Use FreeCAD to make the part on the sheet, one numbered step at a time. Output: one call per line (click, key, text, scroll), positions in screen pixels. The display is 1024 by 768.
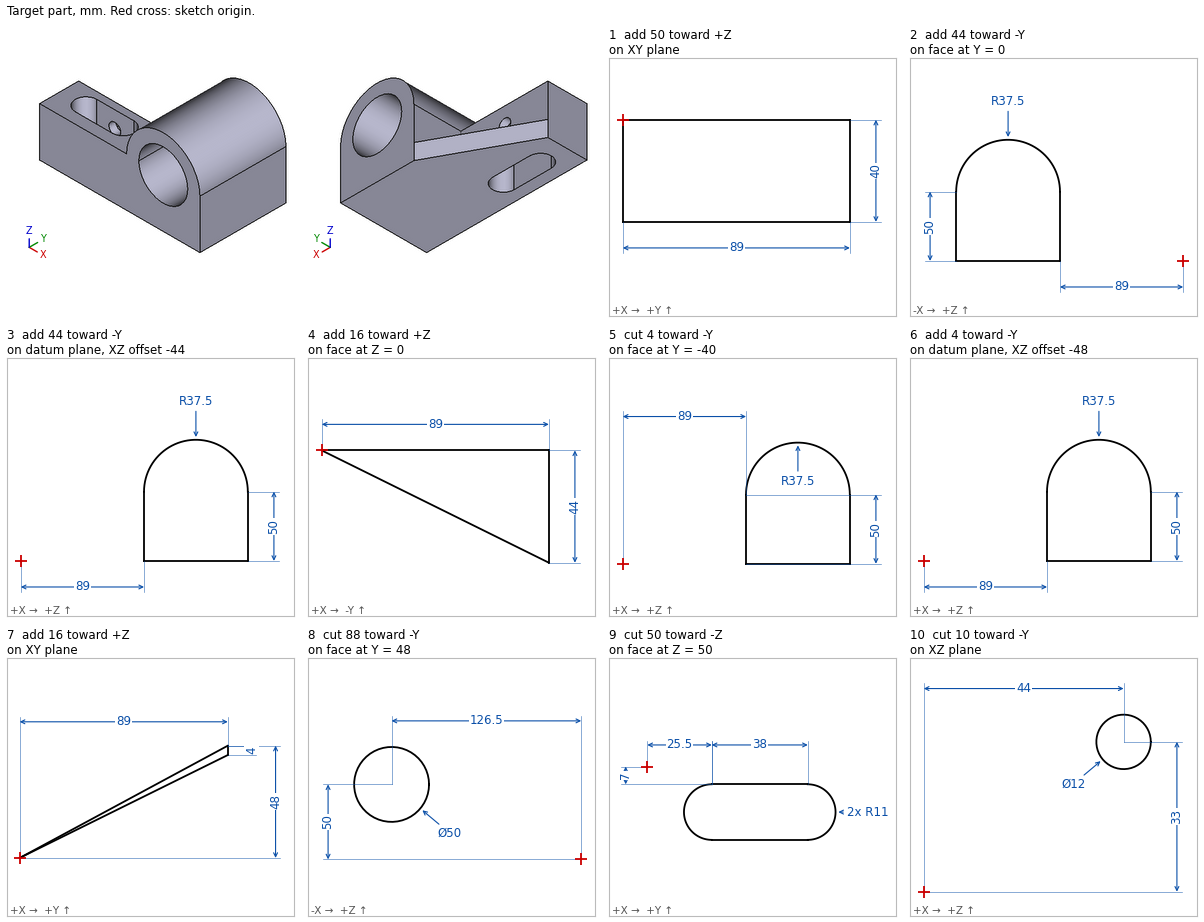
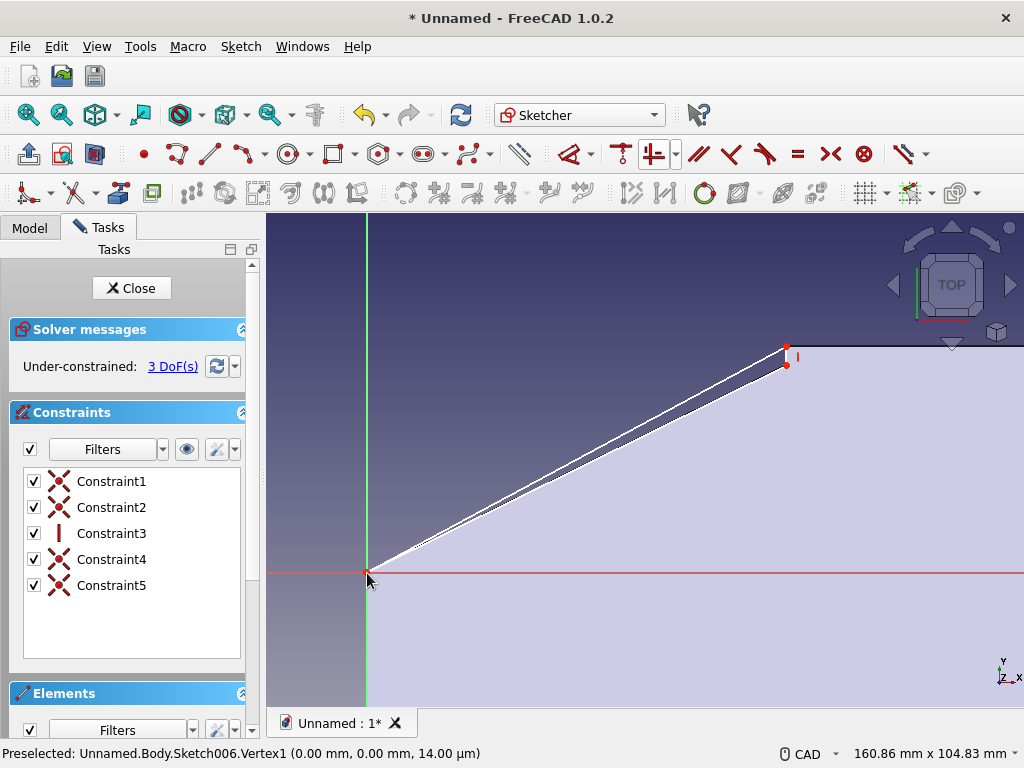
click(568, 154)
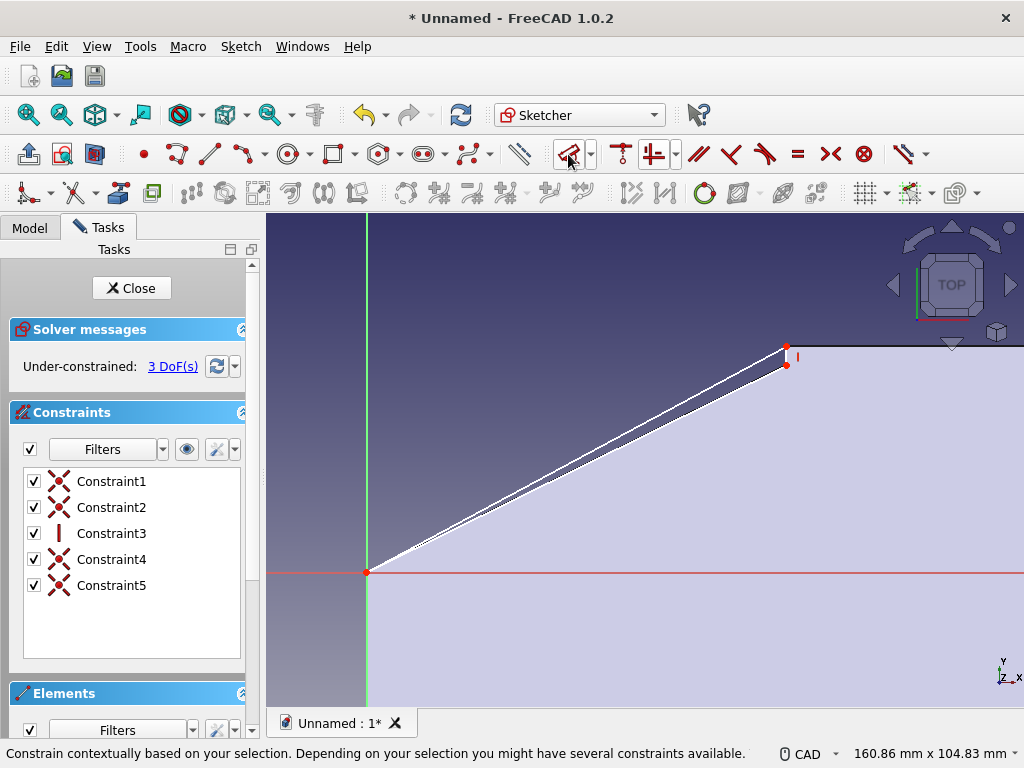
scroll(786, 356, up, 4)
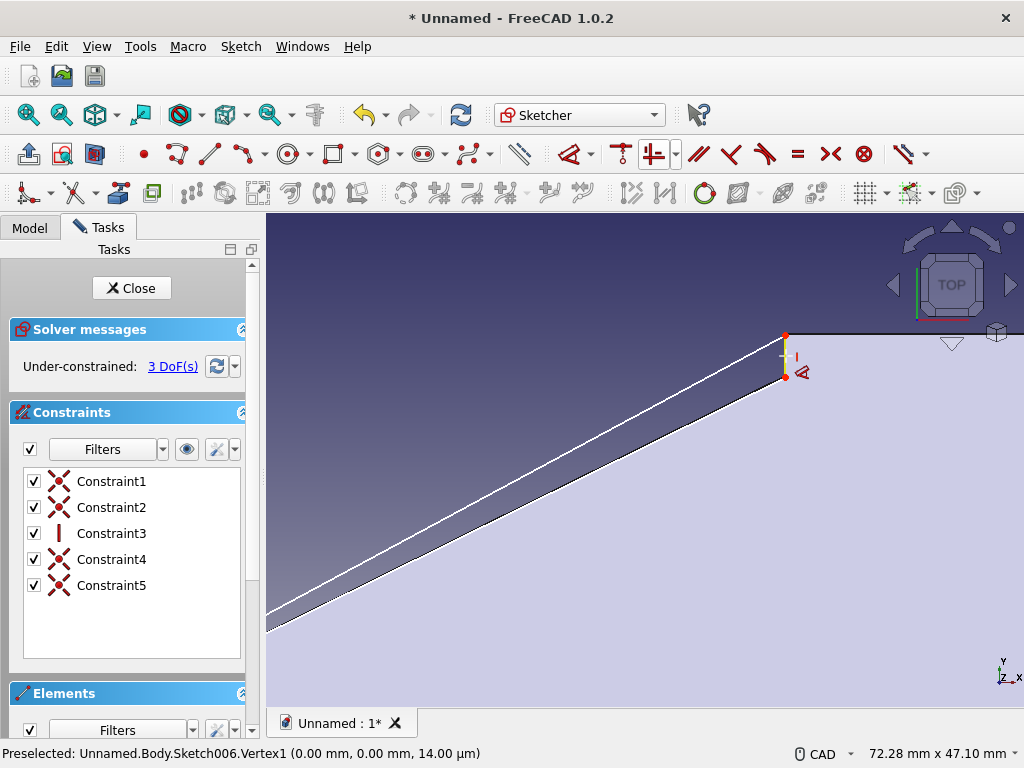
click(785, 357)
click(819, 357)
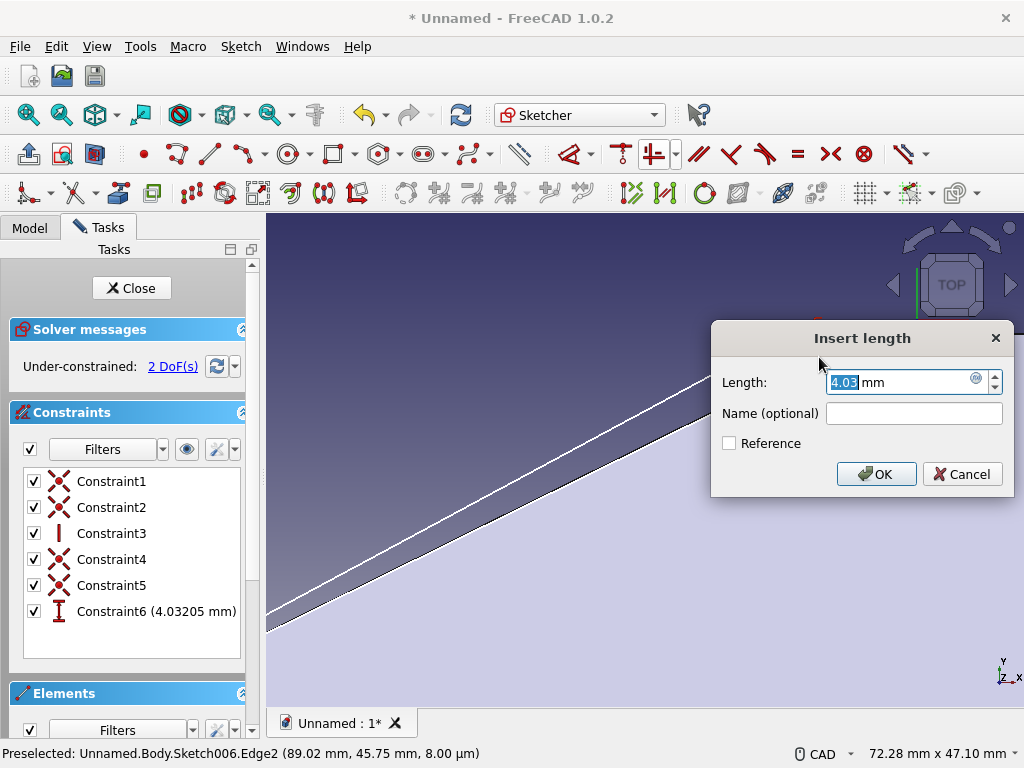
text(4)
key(Return)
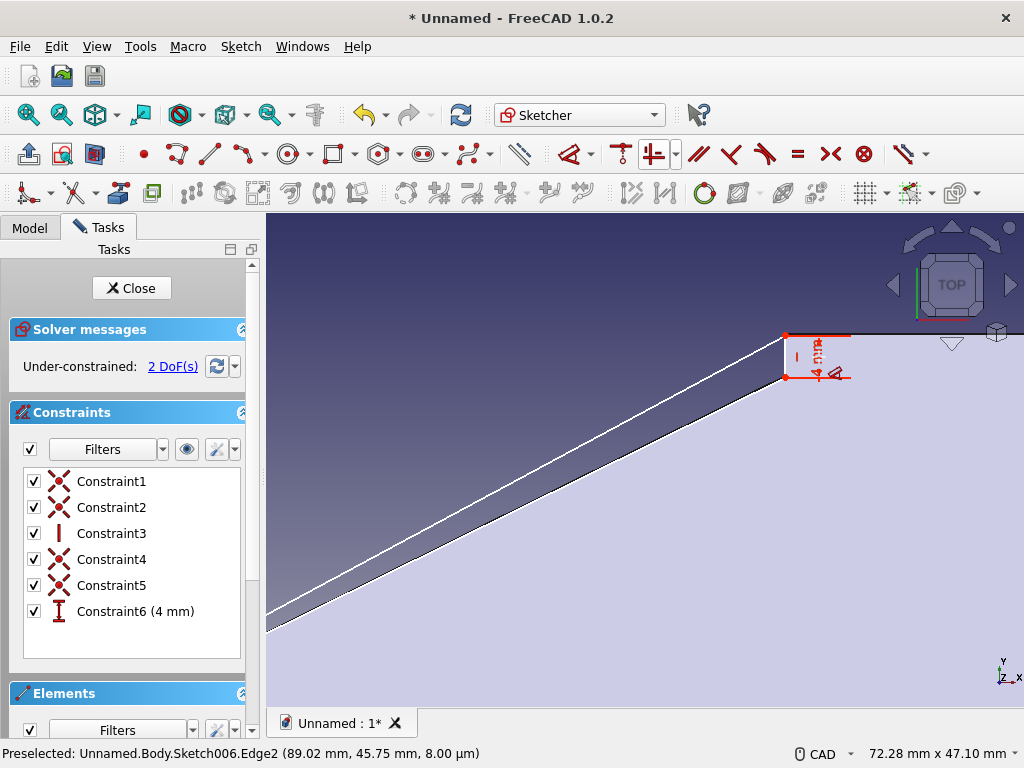
click(785, 336)
click(540, 302)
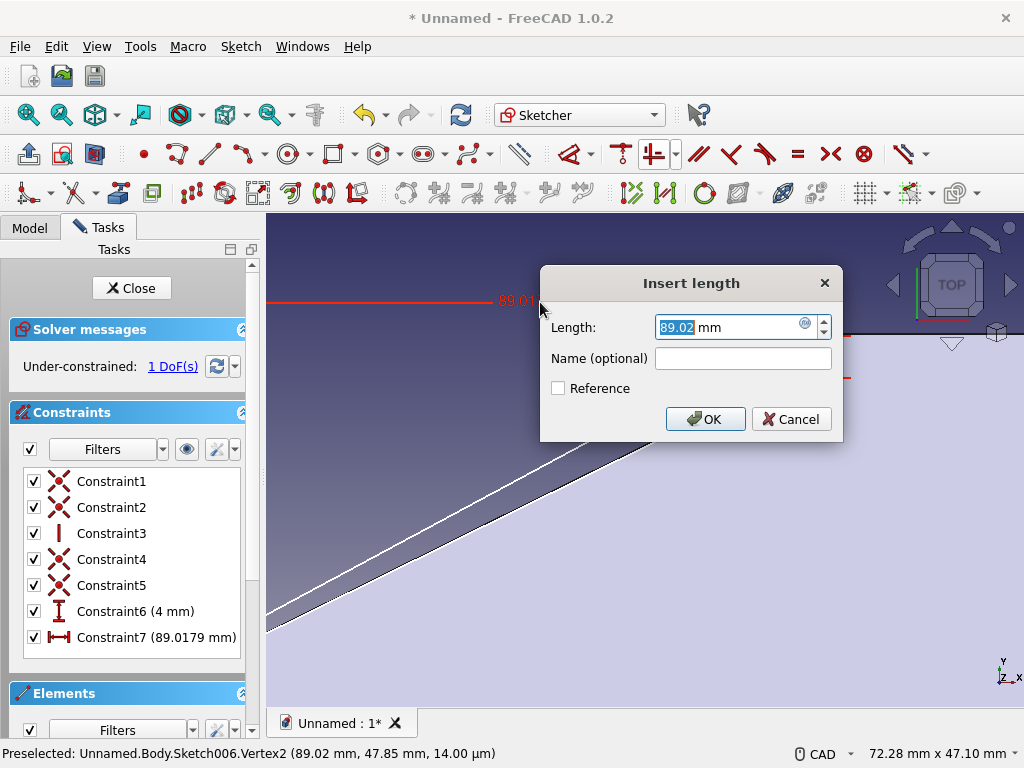
text(89)
key(Return)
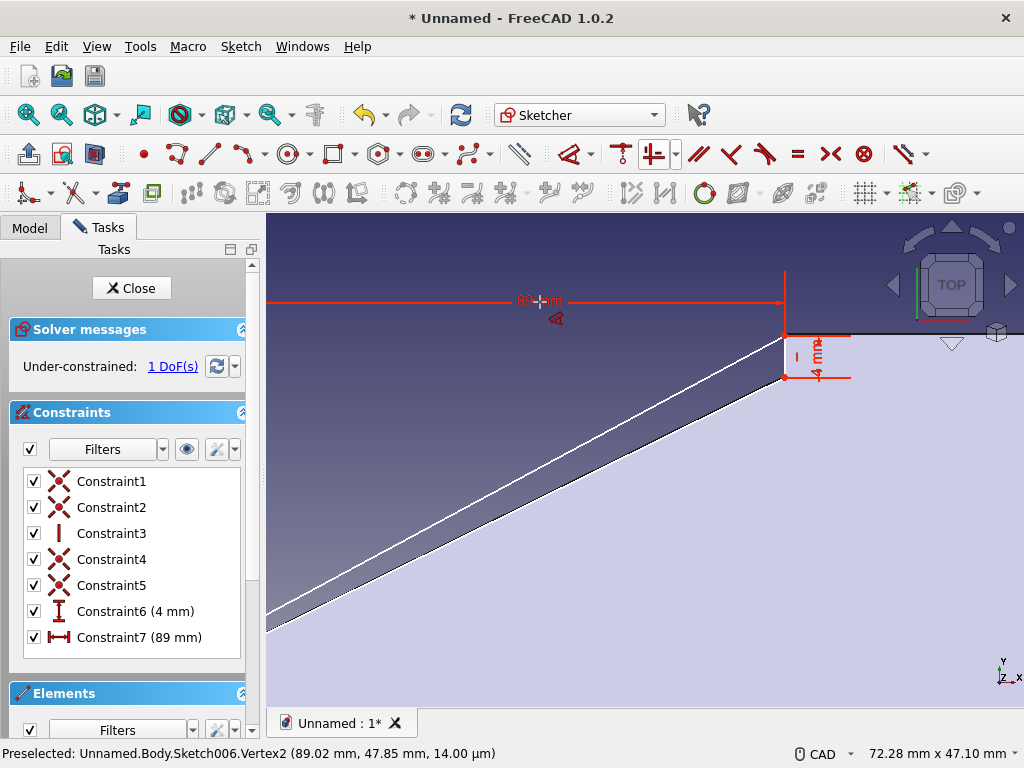
click(785, 336)
click(819, 507)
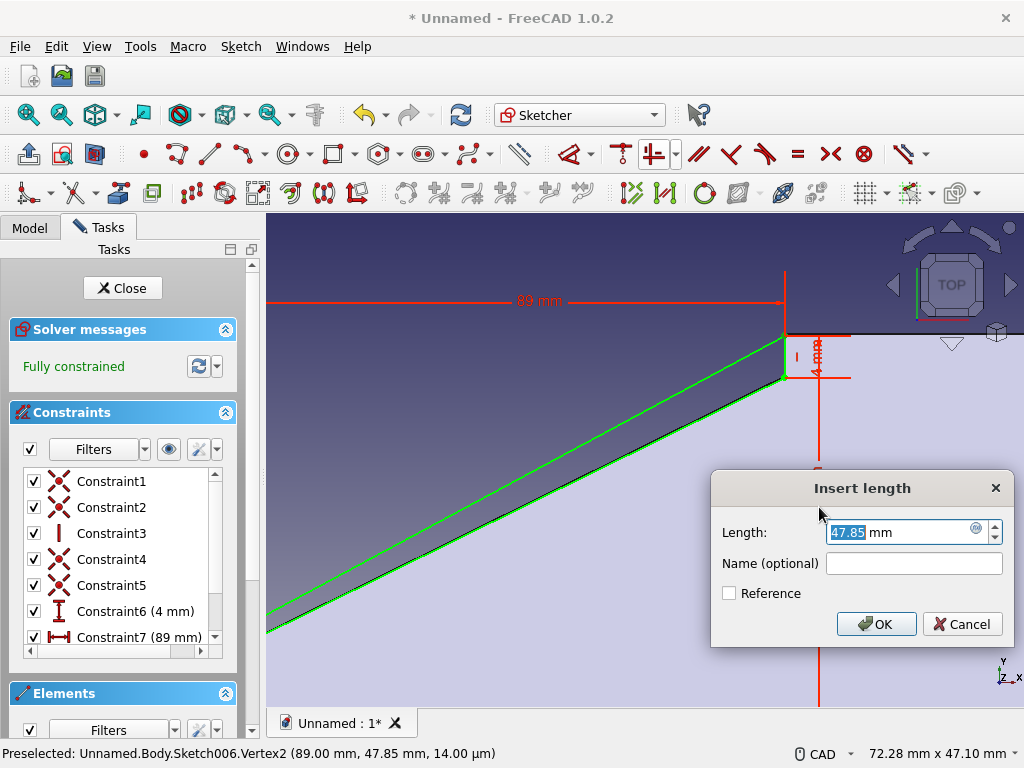
text(48)
key(Return)
key(Escape)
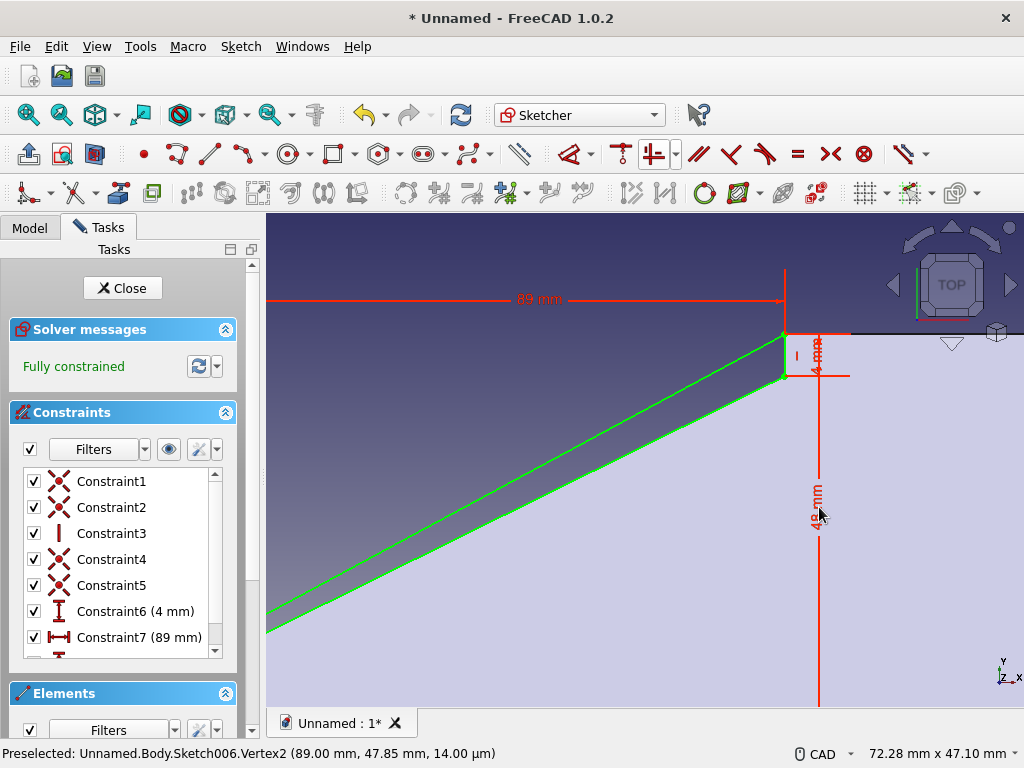
click(123, 288)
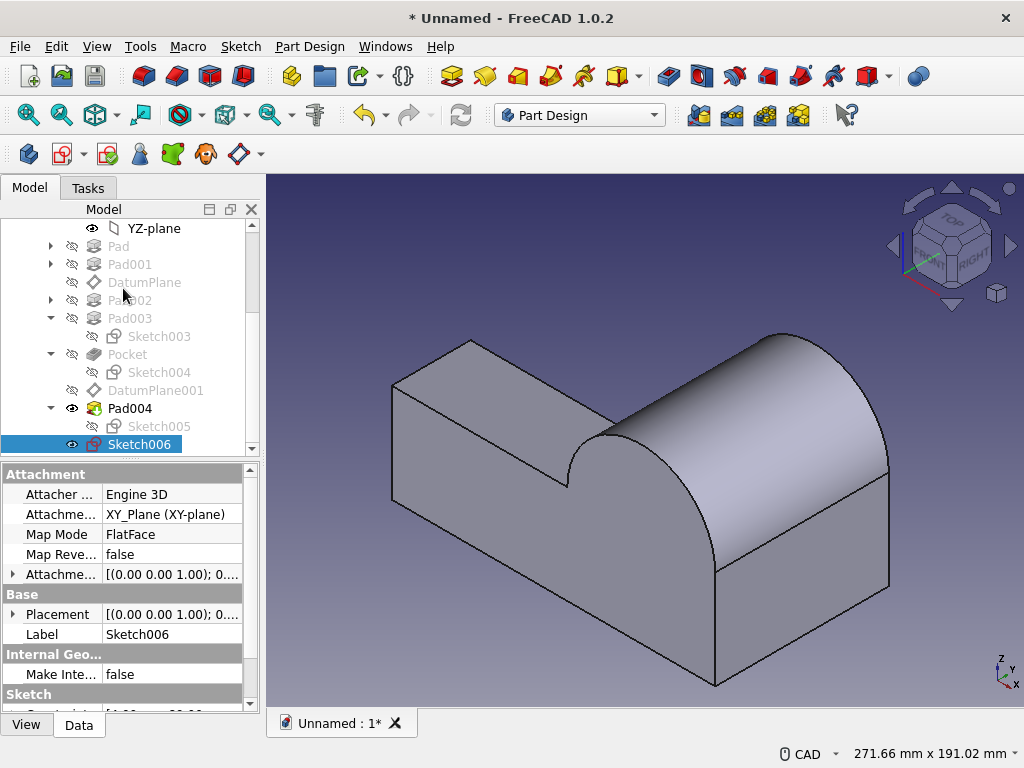
click(452, 76)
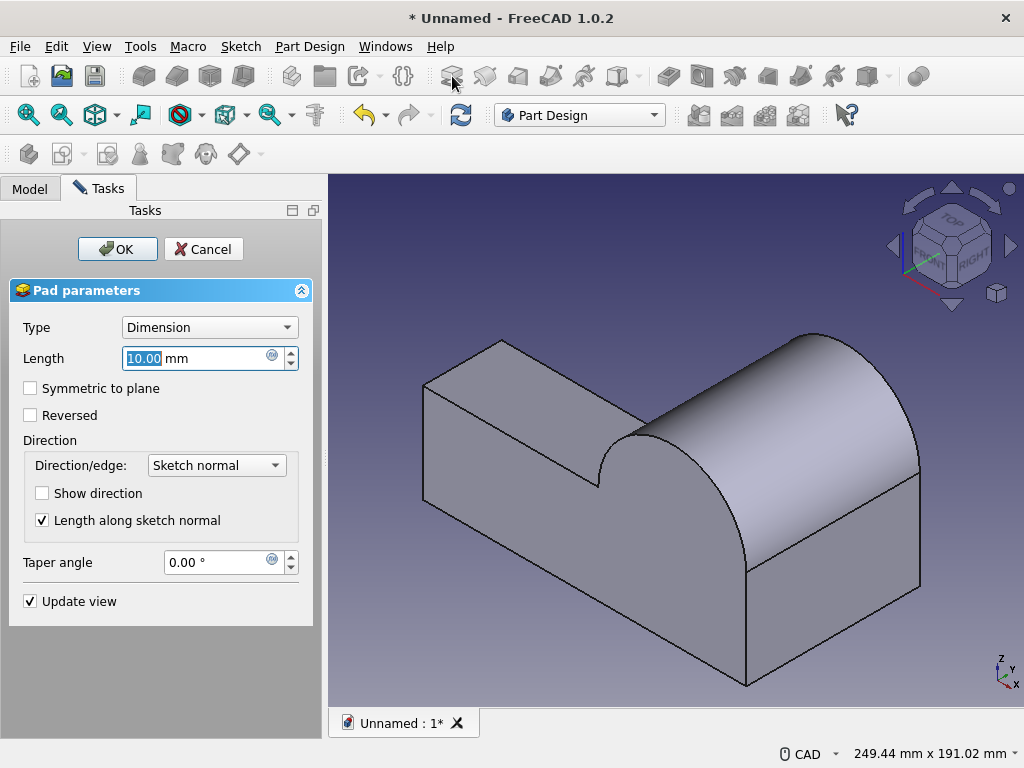
text(16)
key(Tab)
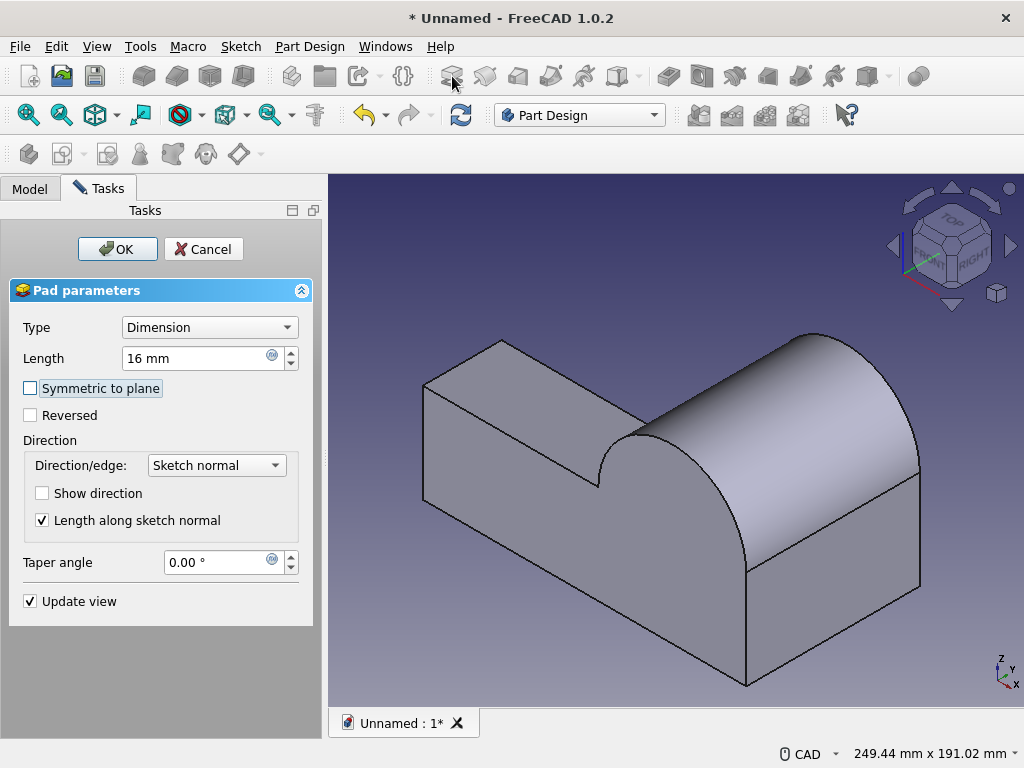
click(118, 249)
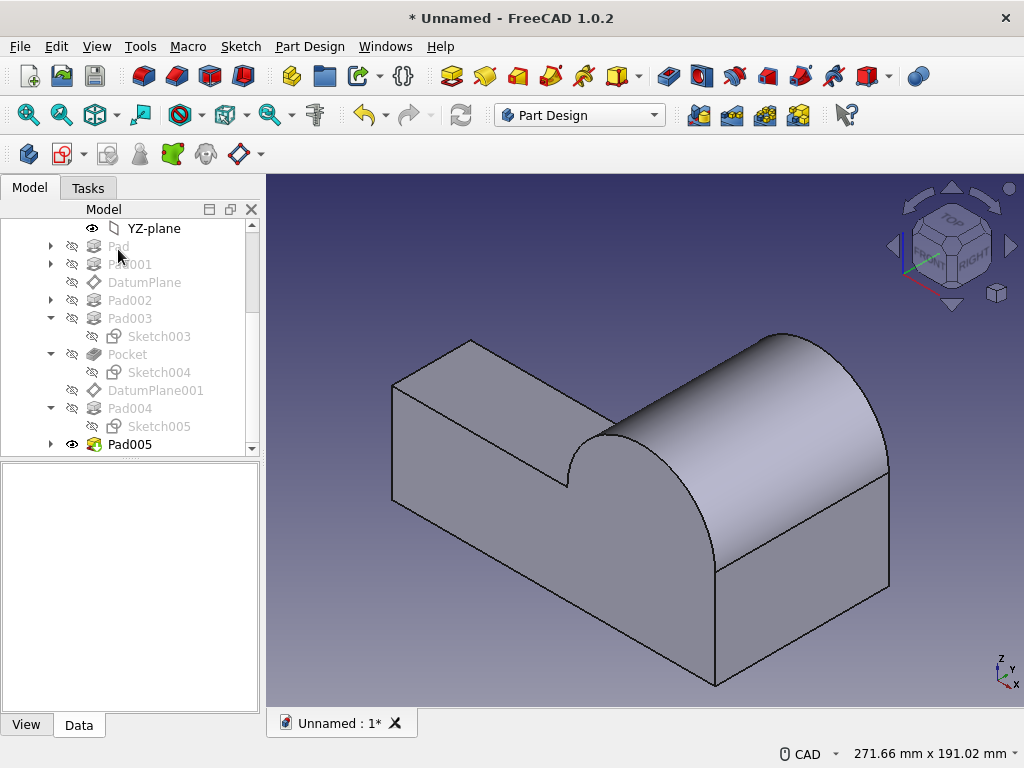
key(4)